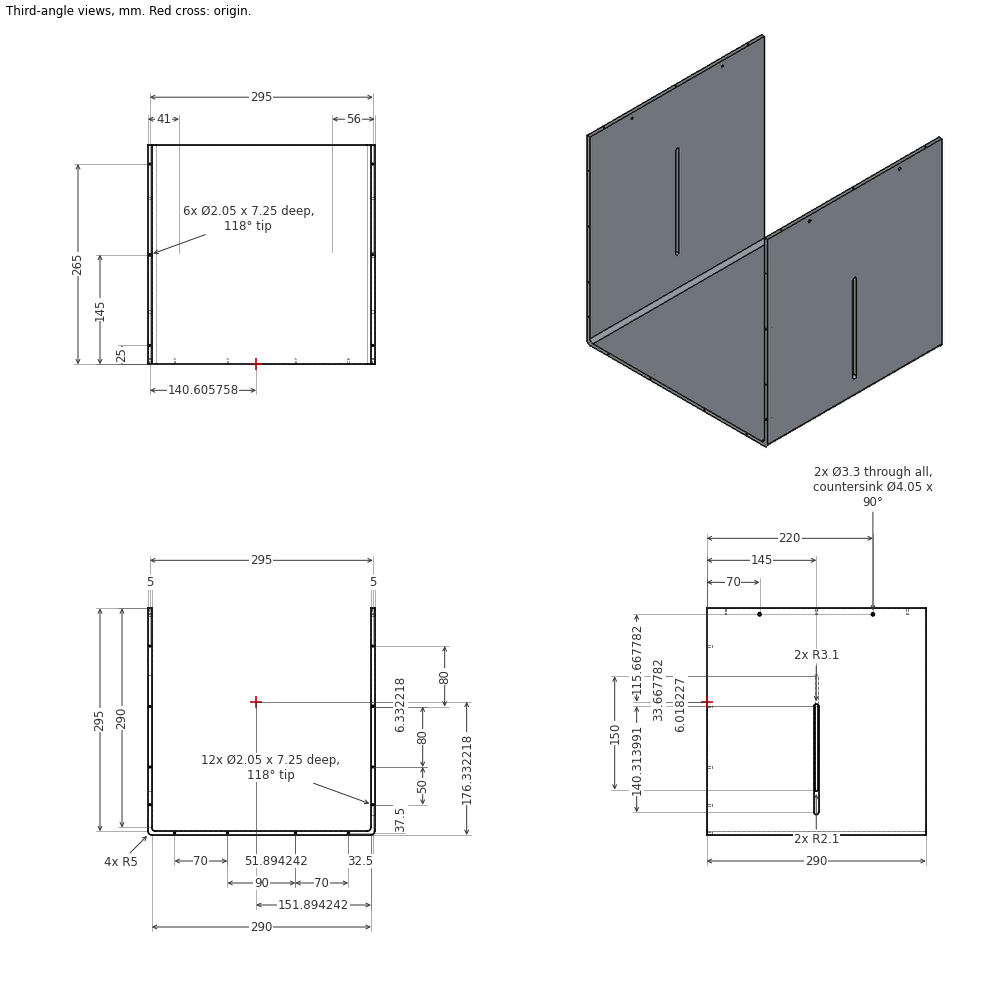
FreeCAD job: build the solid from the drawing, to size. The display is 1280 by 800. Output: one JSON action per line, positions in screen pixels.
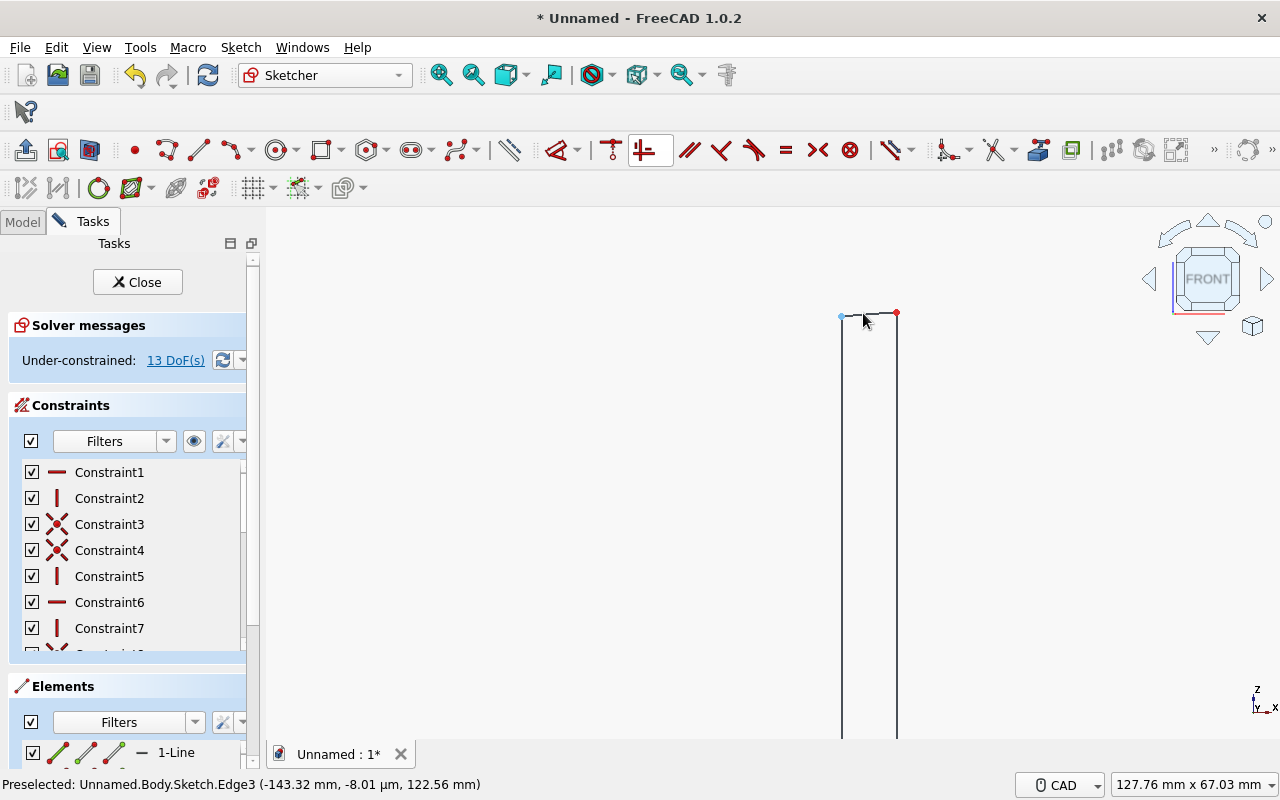
{"action": "left_click", "coordinate": [858, 315]}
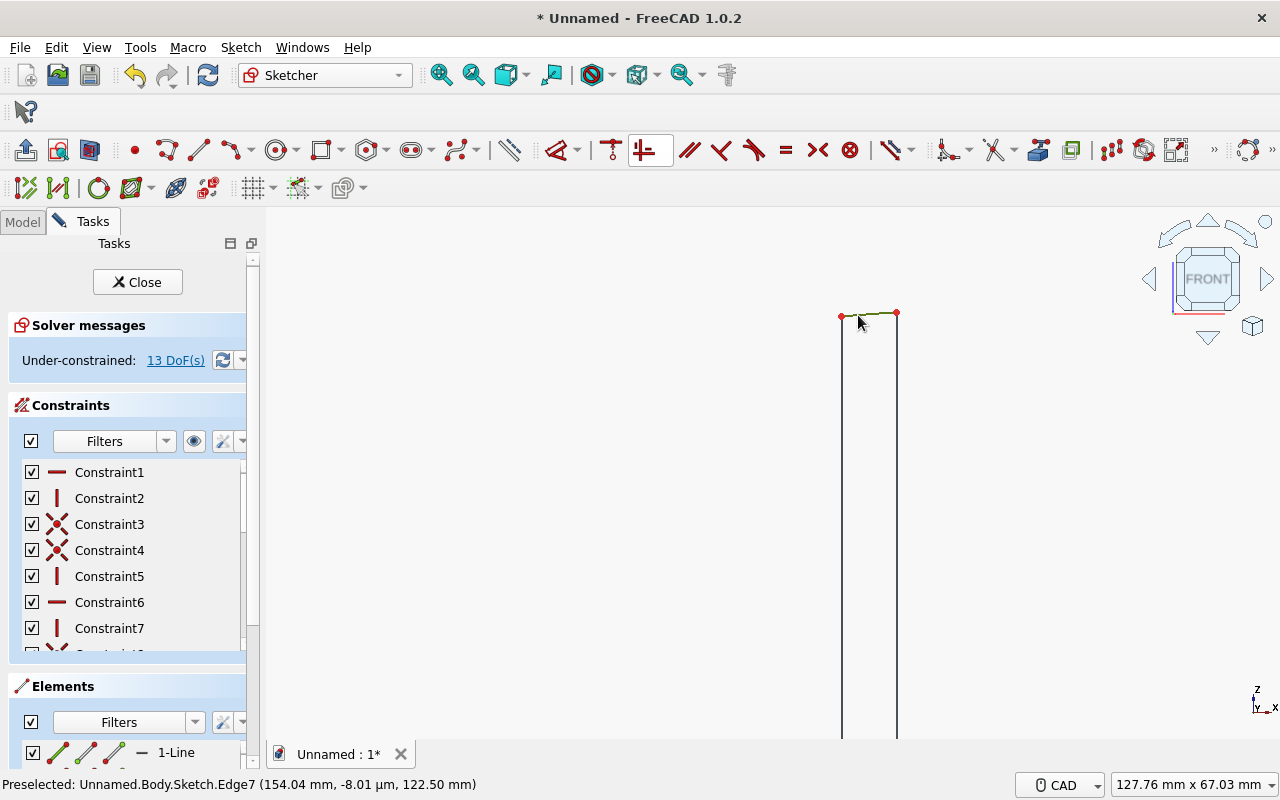
{"action": "key", "text": "h"}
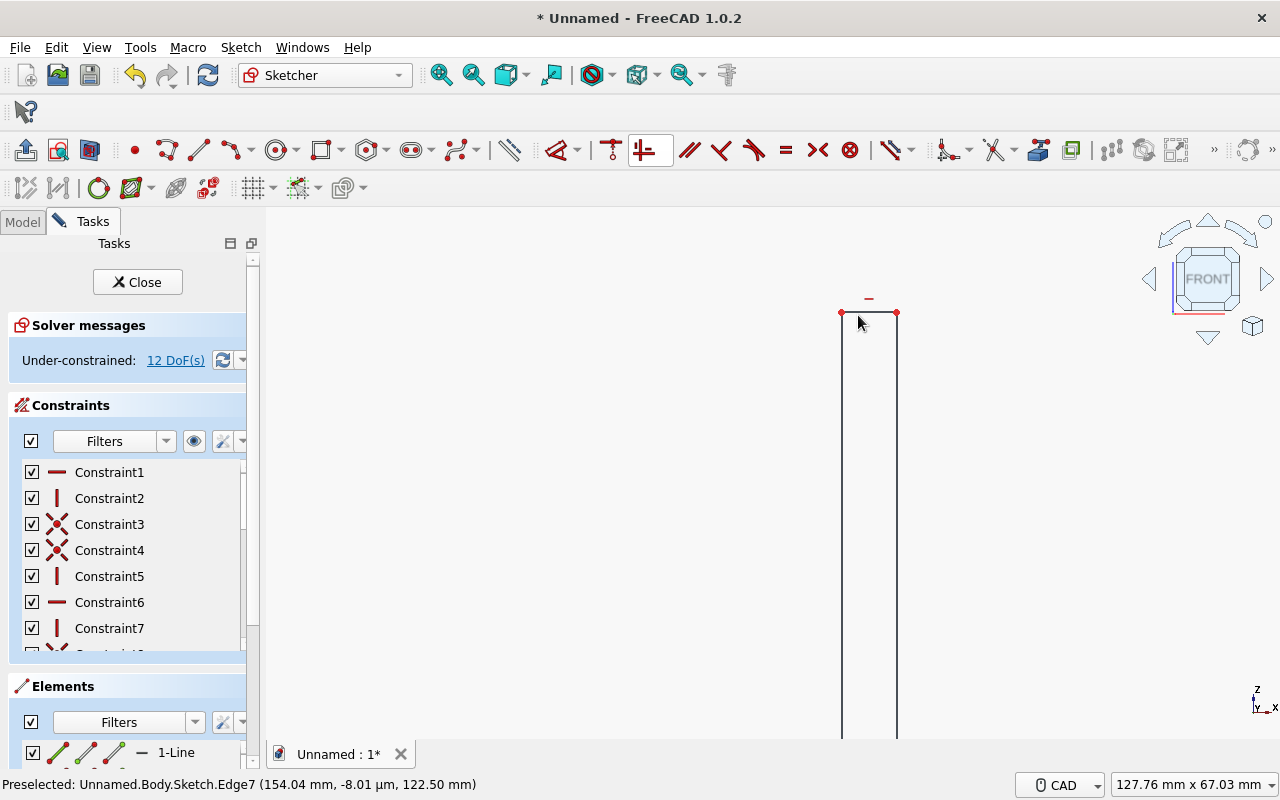
{"action": "scroll", "coordinate": [863, 313], "scroll_direction": "down", "scroll_amount": 10}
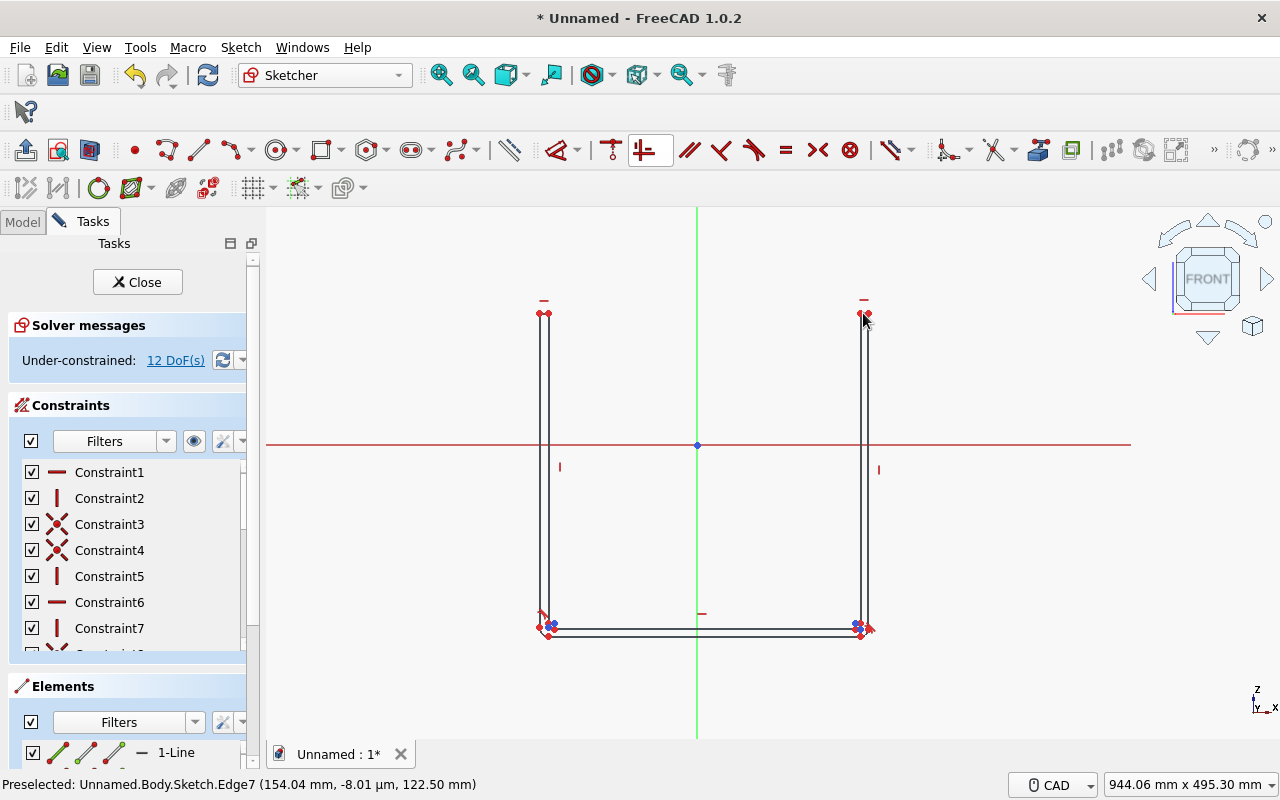
{"action": "scroll", "coordinate": [541, 632], "scroll_direction": "up", "scroll_amount": 6}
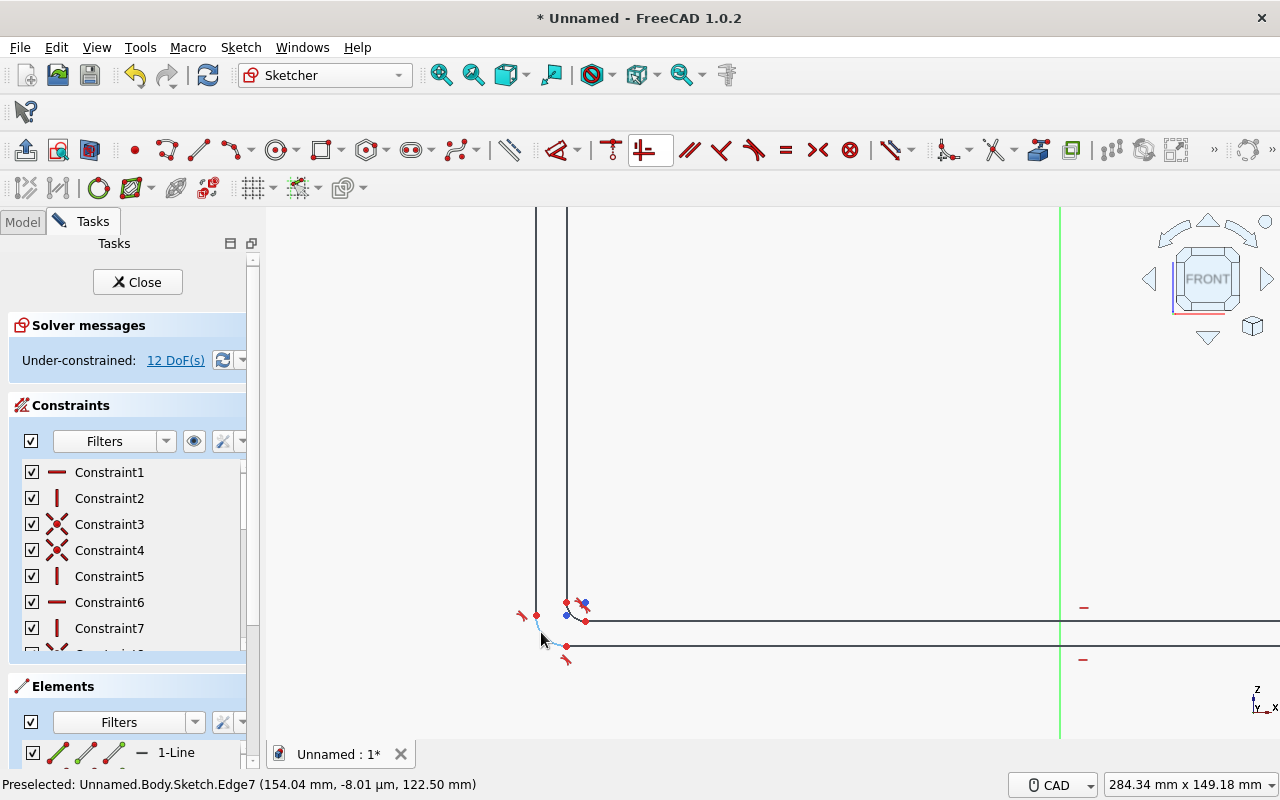
{"action": "left_click", "coordinate": [539, 629]}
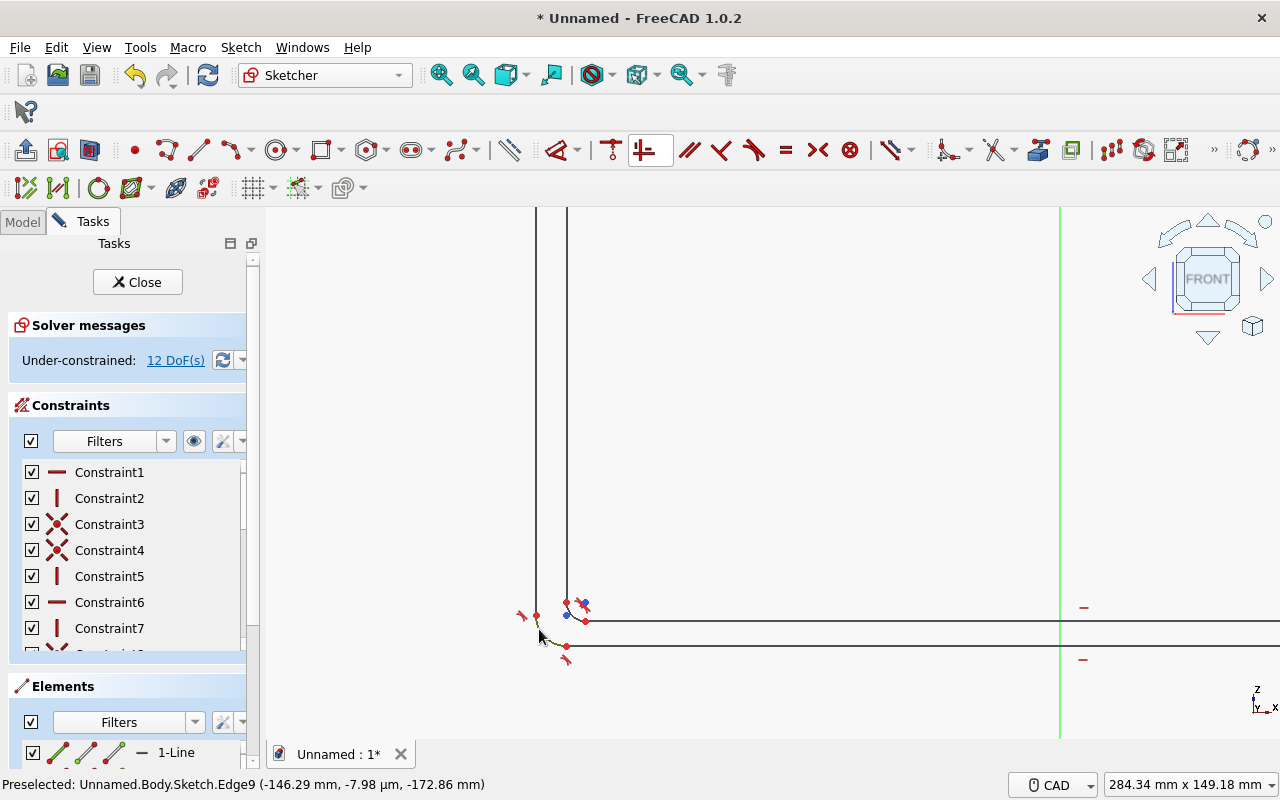
{"action": "left_click", "coordinate": [572, 616]}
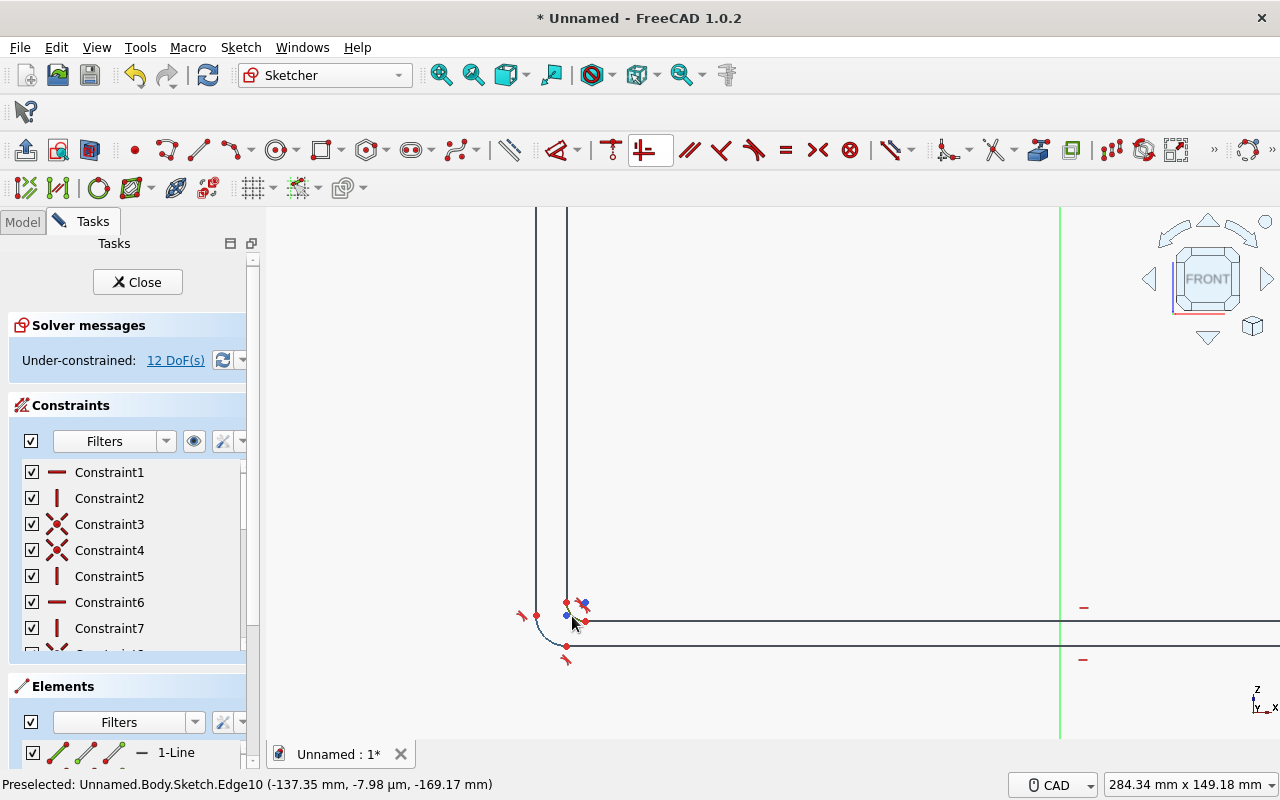
{"action": "scroll", "coordinate": [541, 632], "scroll_direction": "down", "scroll_amount": 6}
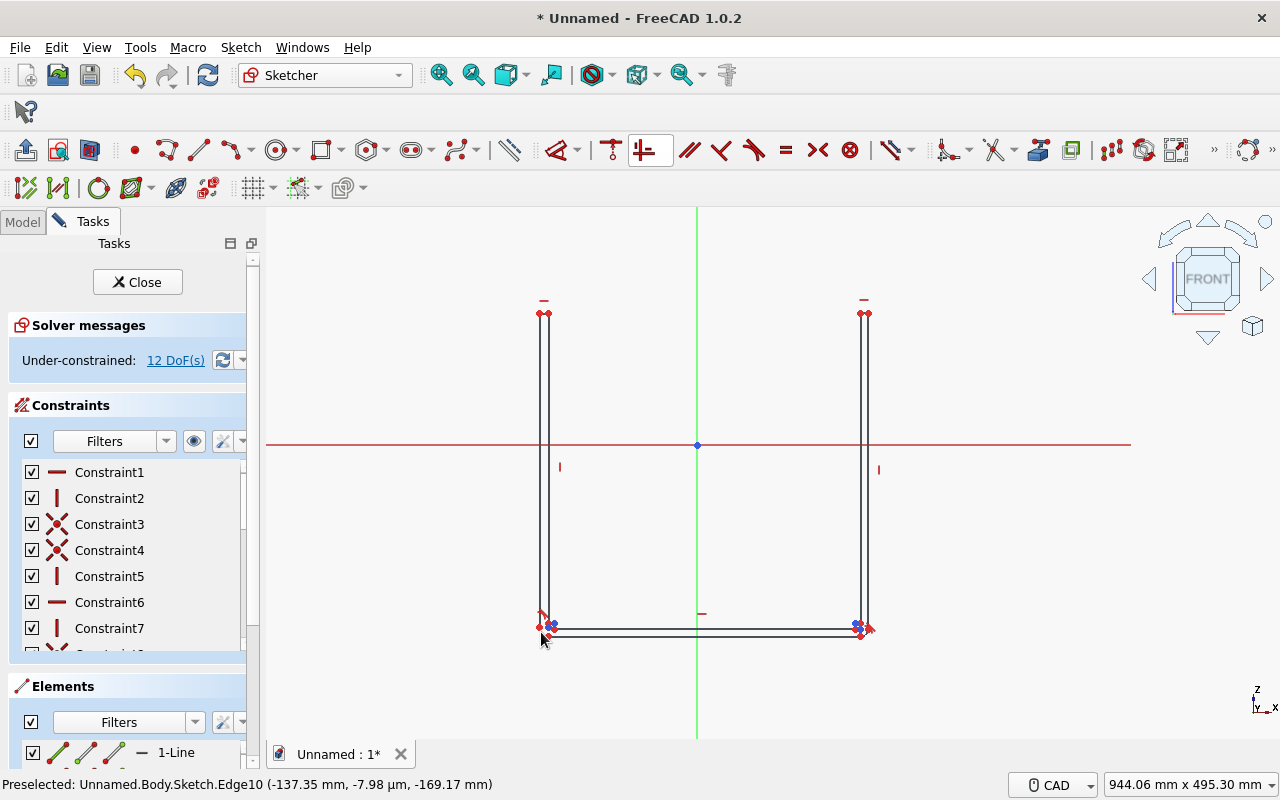
{"action": "scroll", "coordinate": [859, 628], "scroll_direction": "up", "scroll_amount": 7}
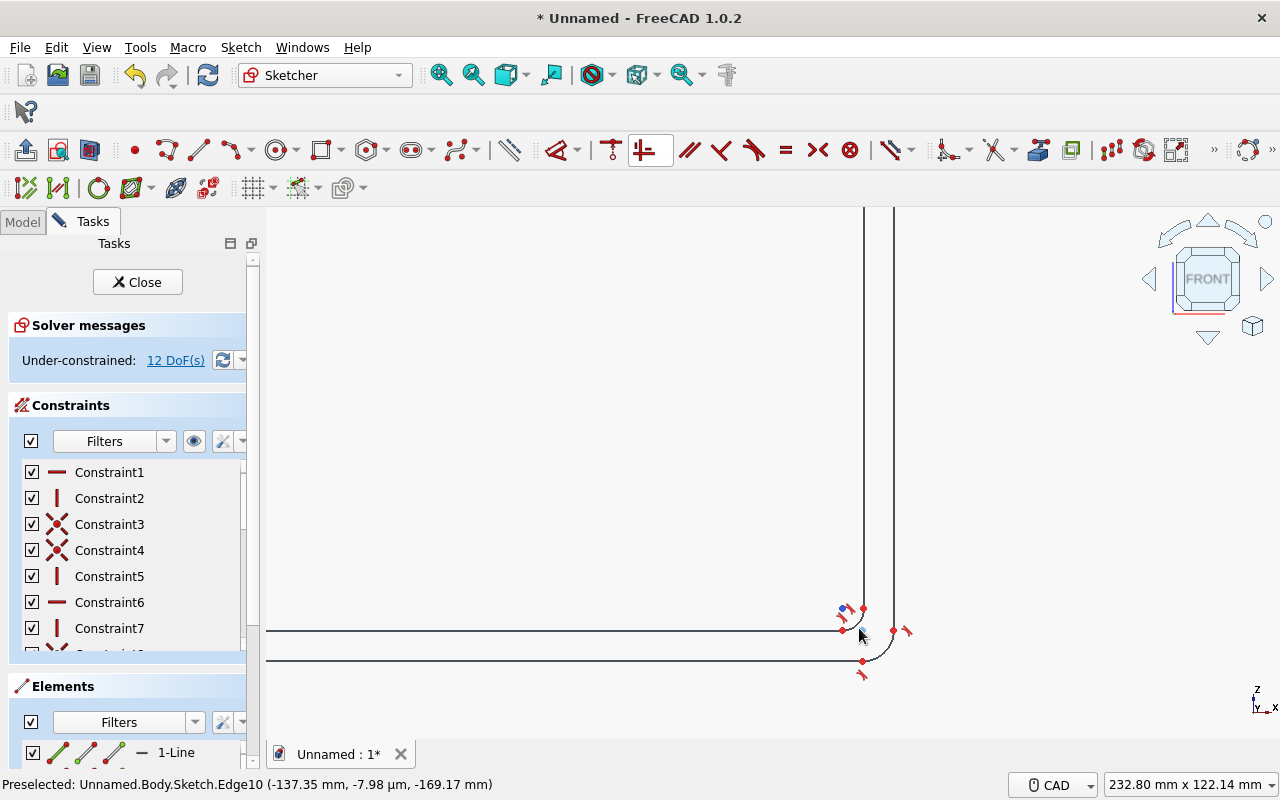
{"action": "left_click", "coordinate": [858, 624]}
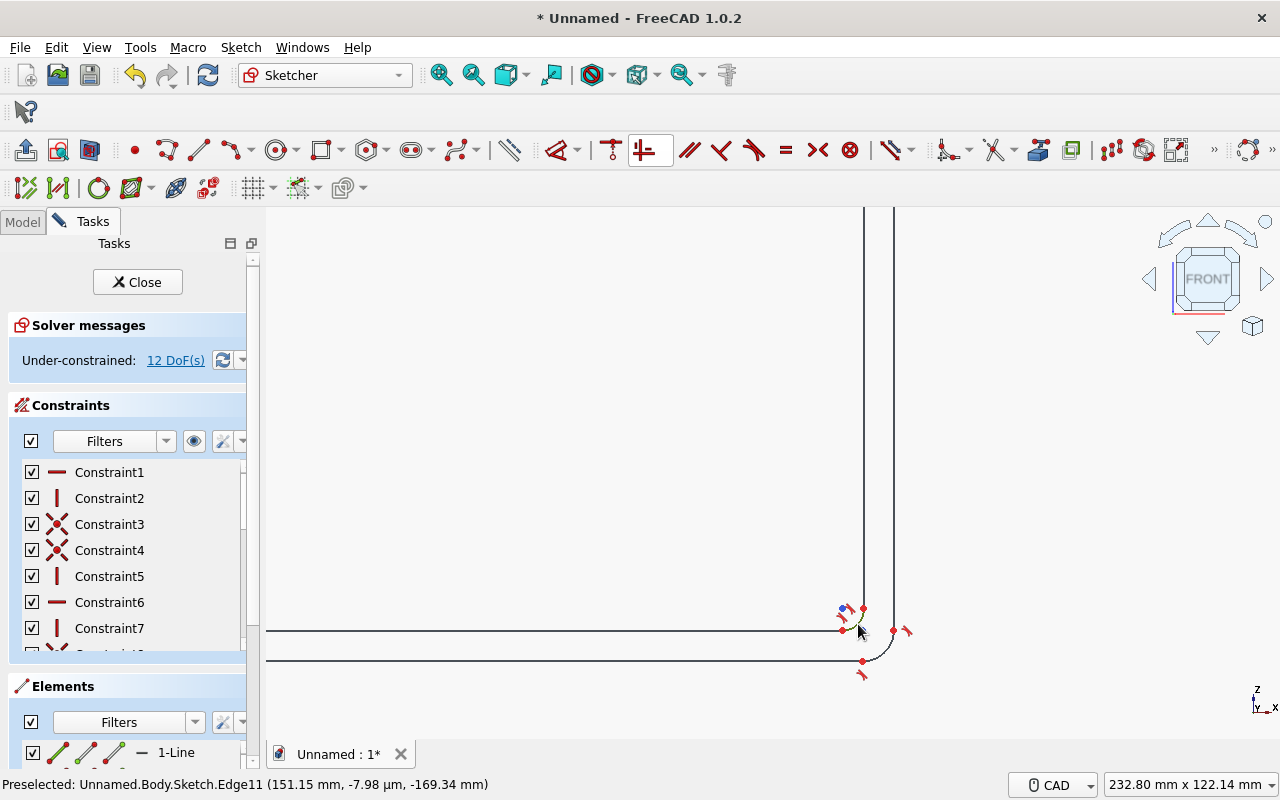
{"action": "left_click", "coordinate": [877, 658]}